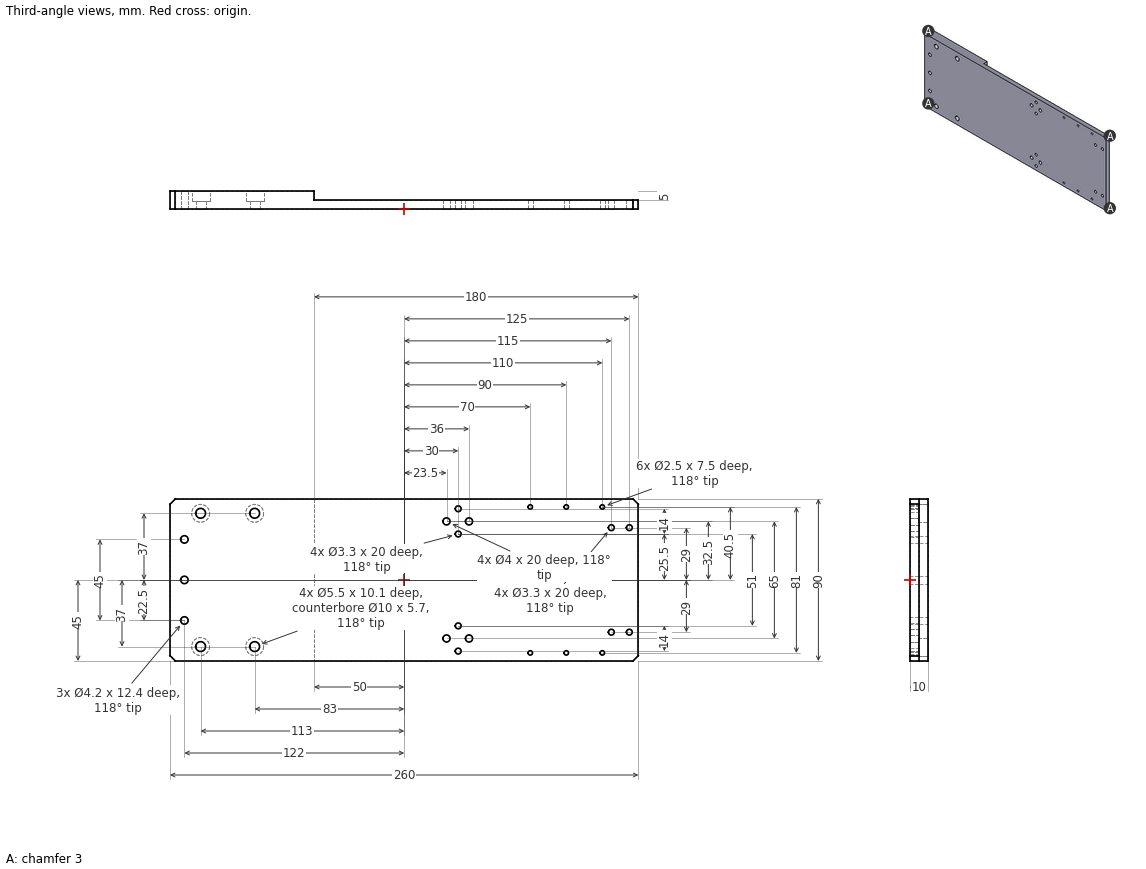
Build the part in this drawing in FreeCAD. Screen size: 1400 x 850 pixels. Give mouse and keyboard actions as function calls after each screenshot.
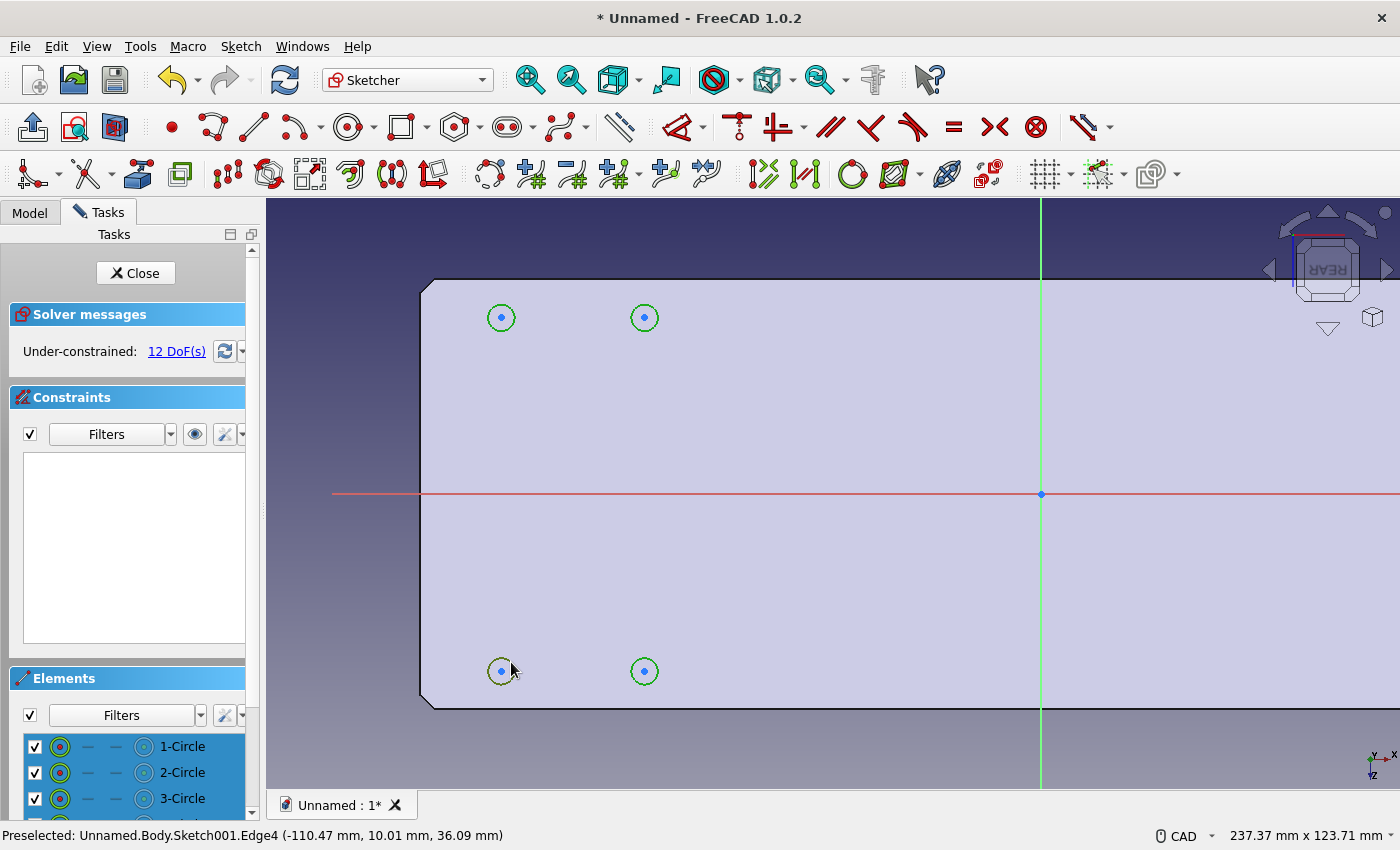
click(954, 128)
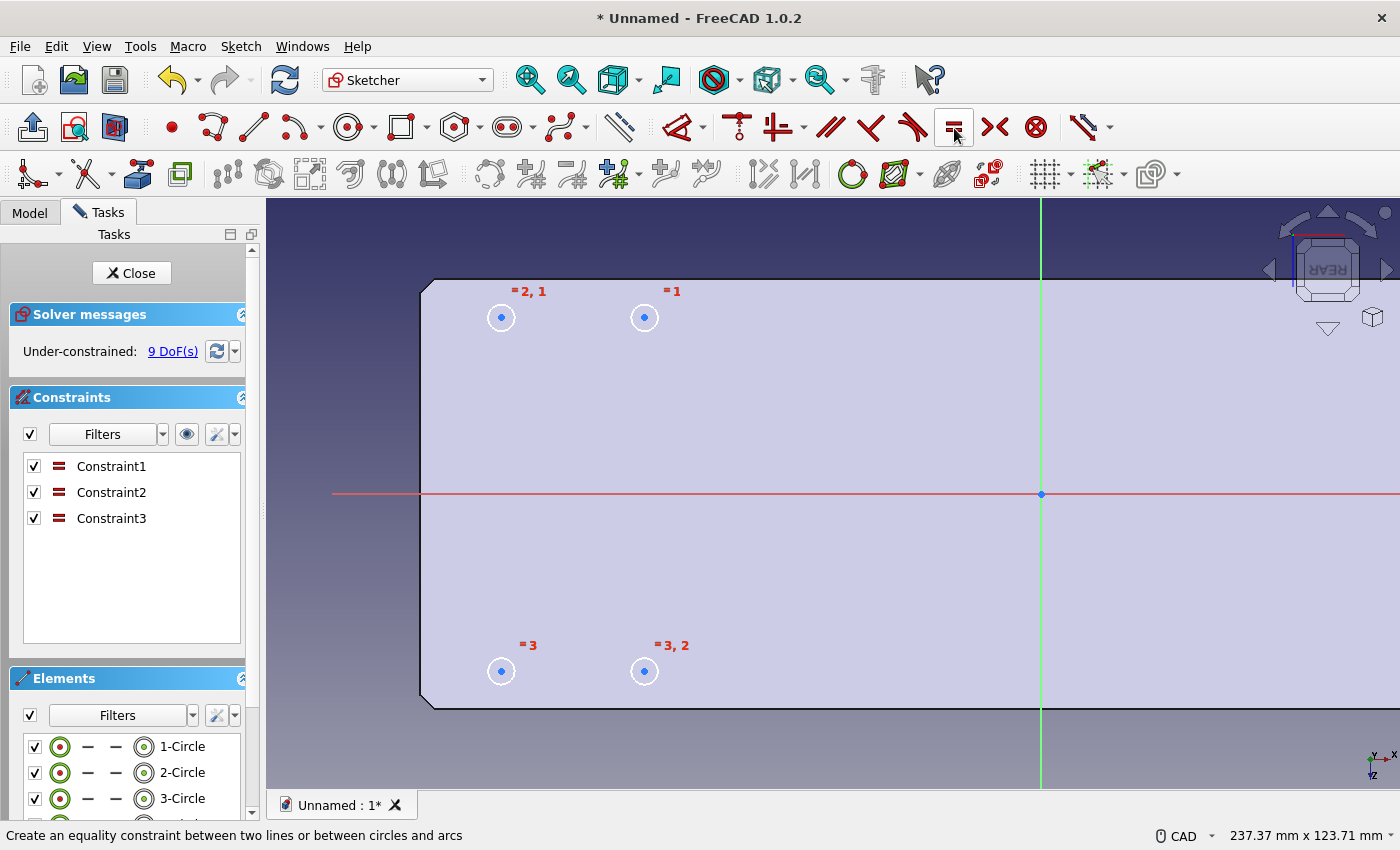
click(645, 318)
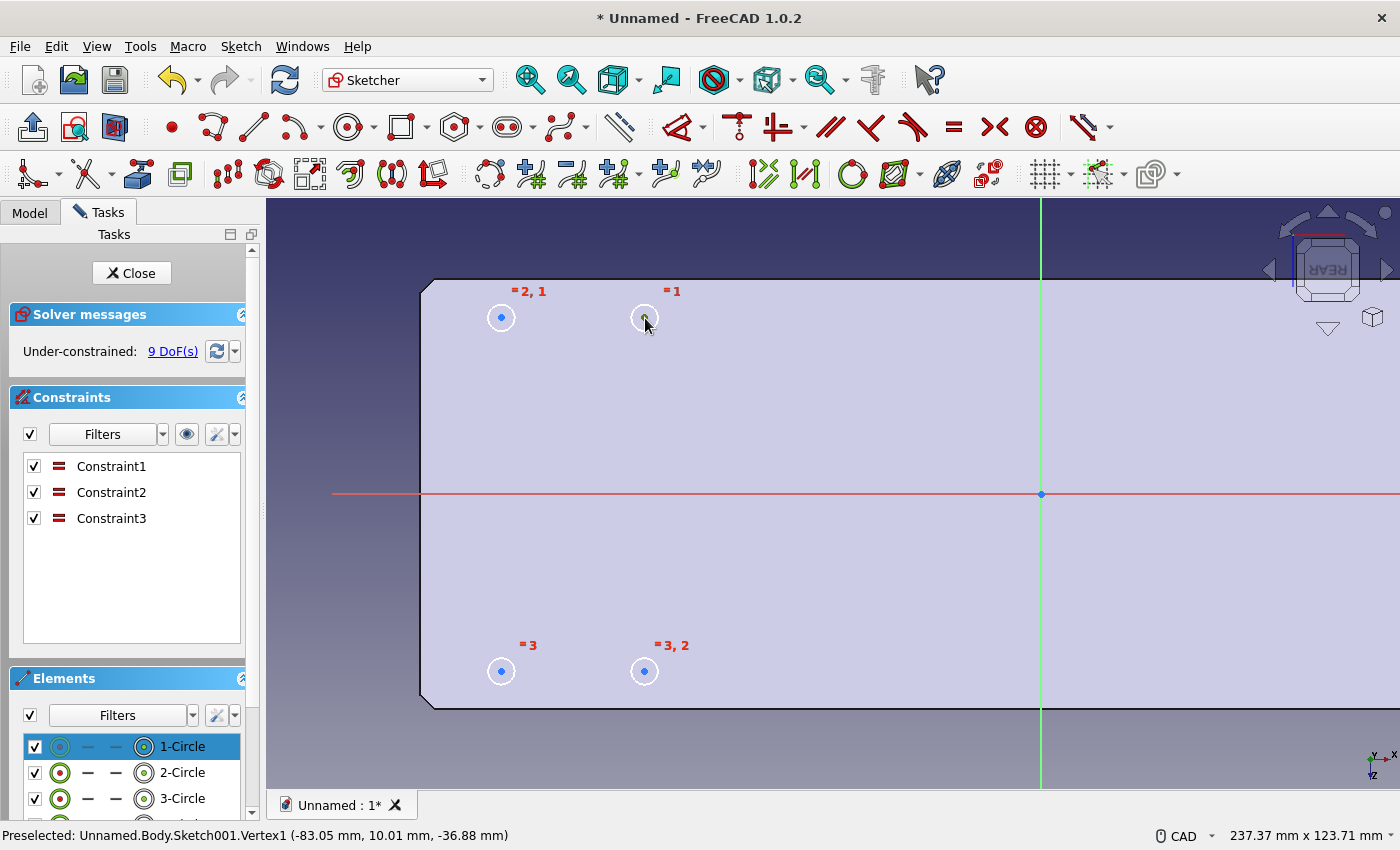
click(501, 318)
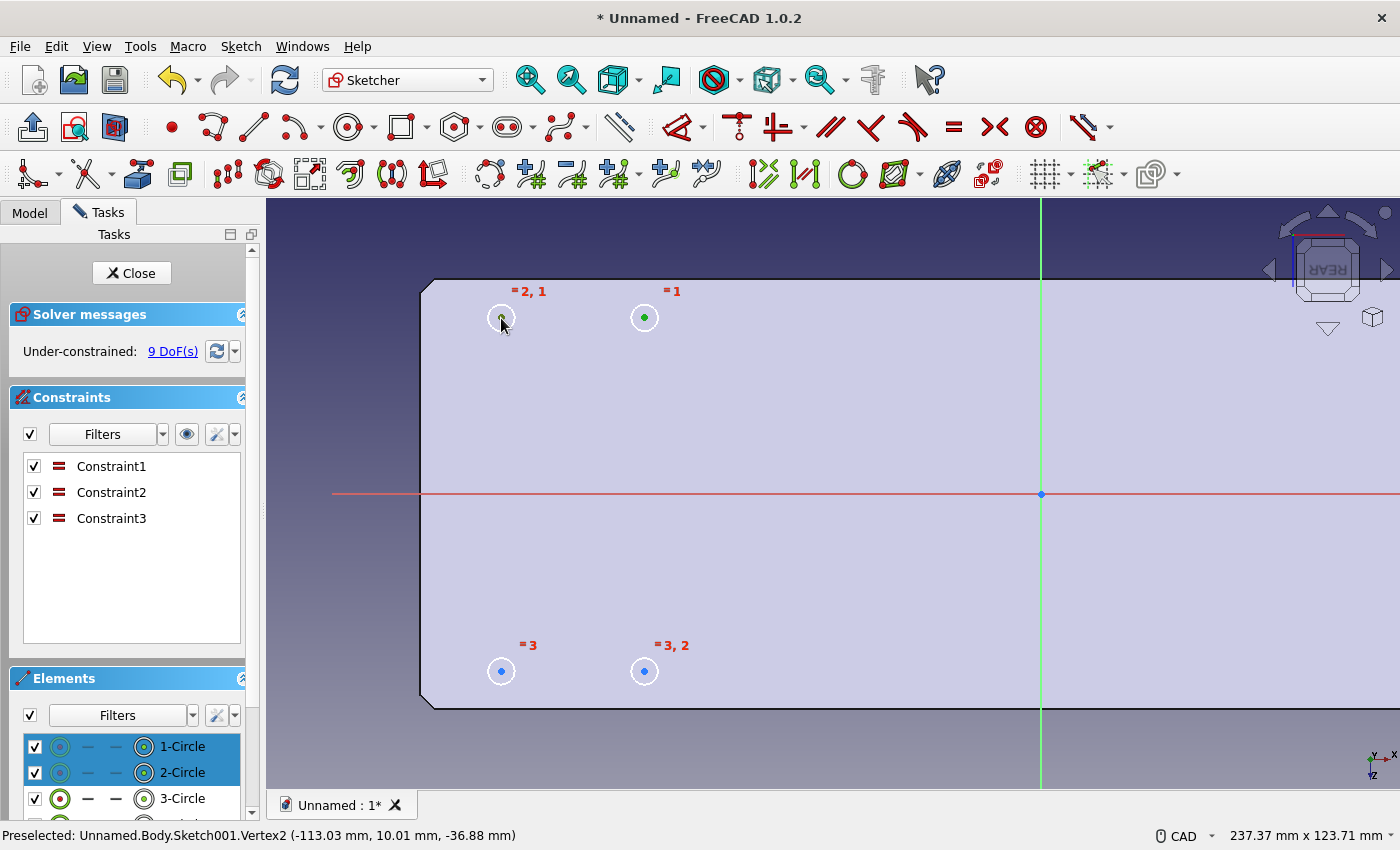
click(804, 128)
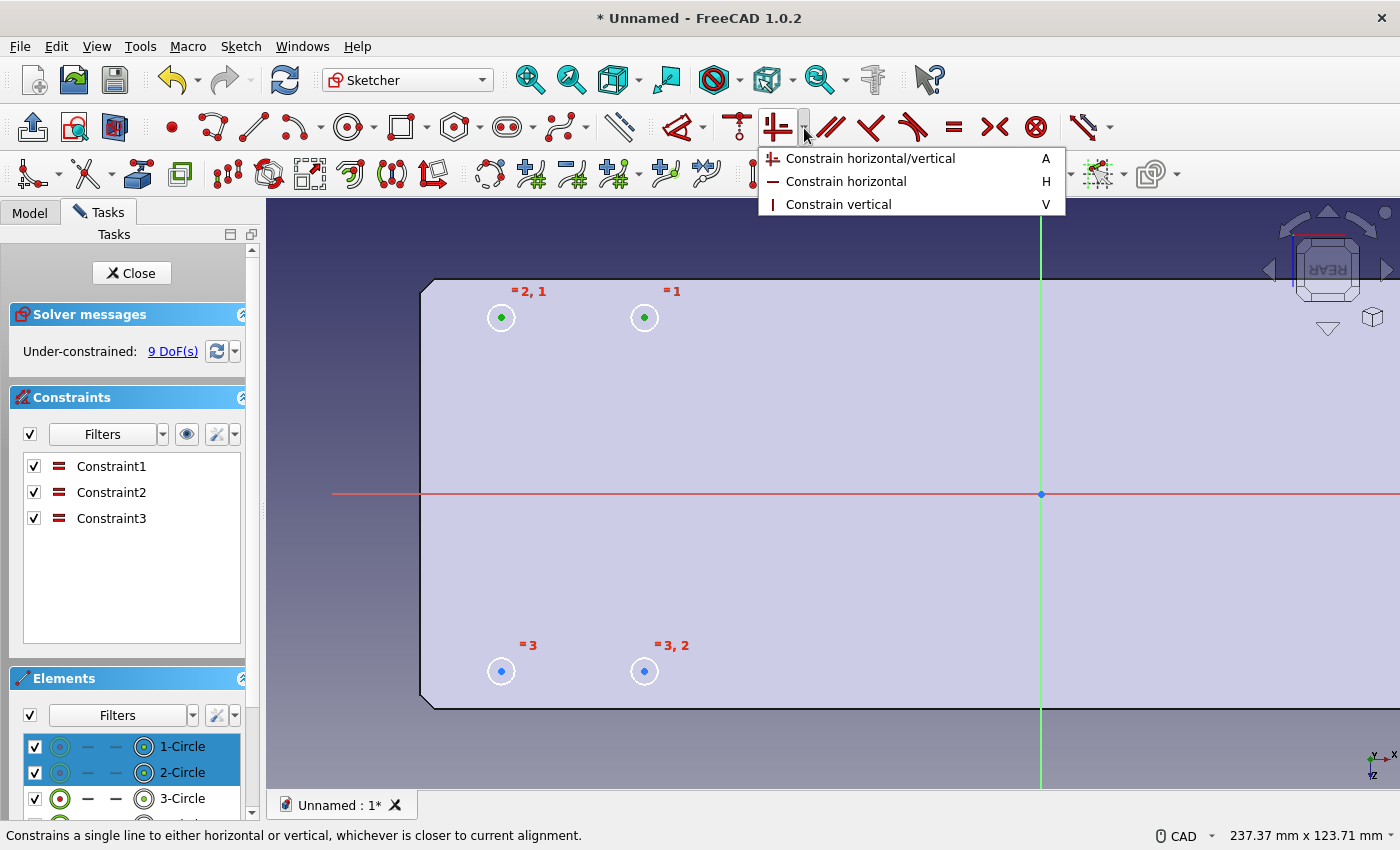
click(912, 182)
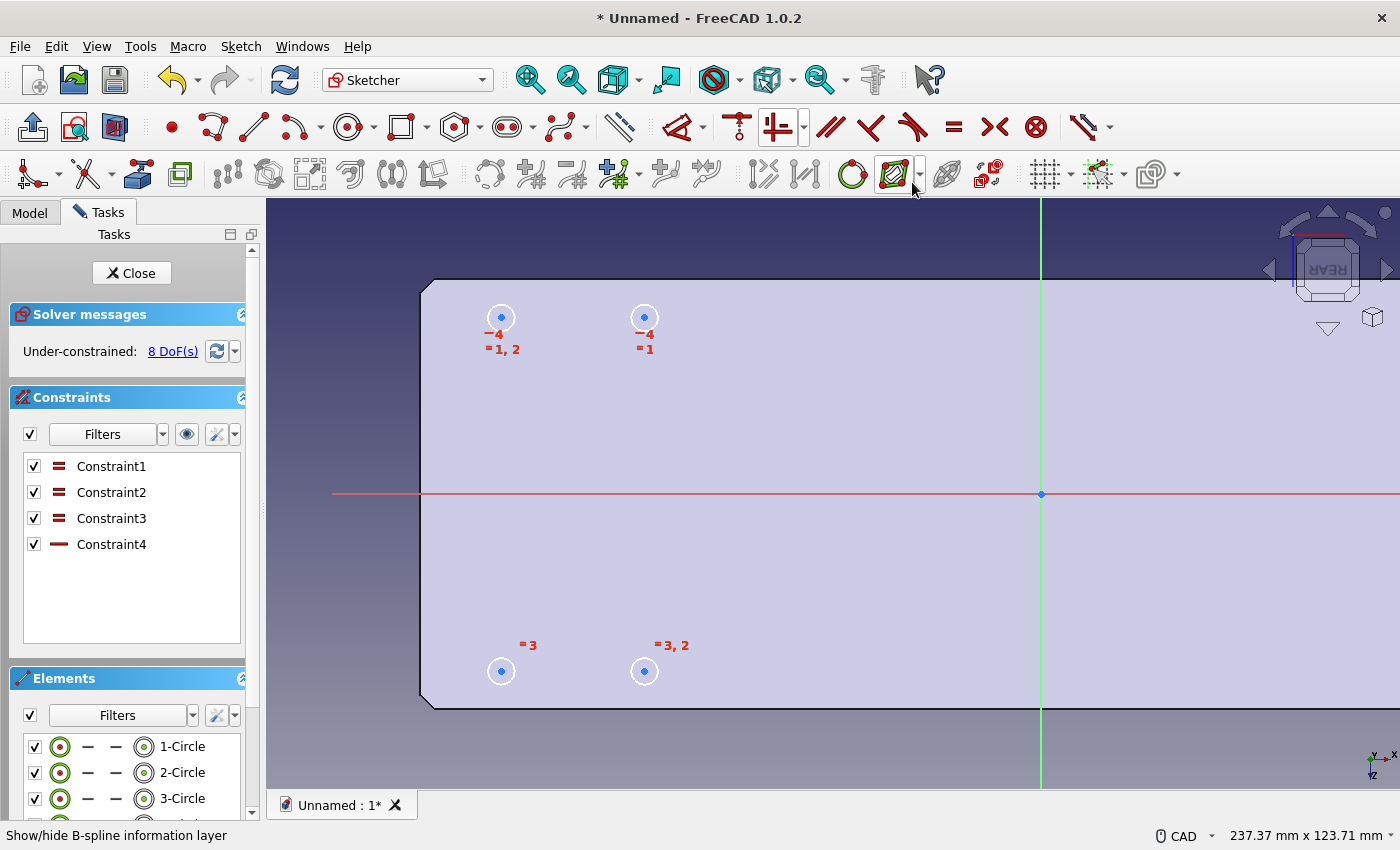
click(645, 318)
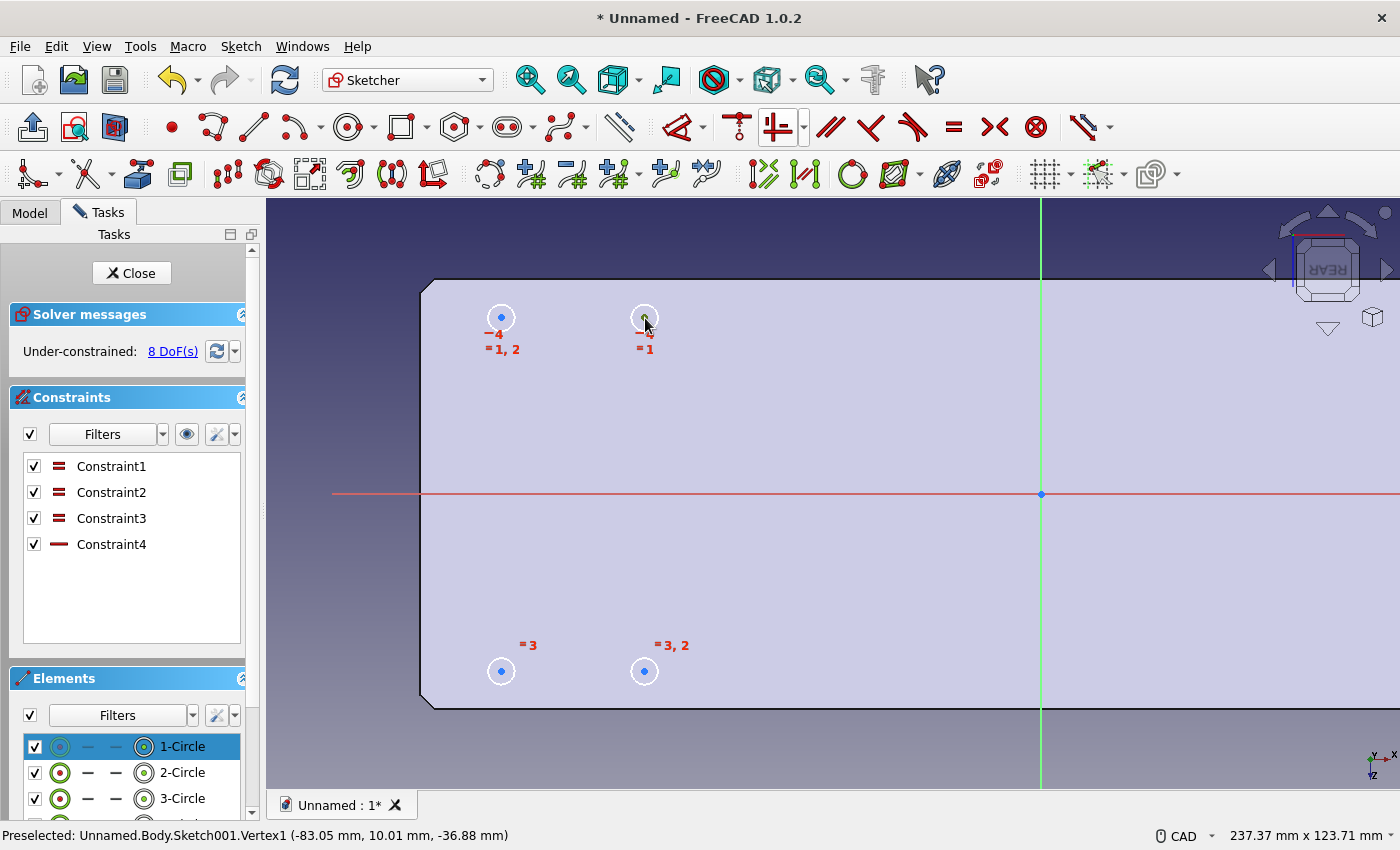
click(645, 671)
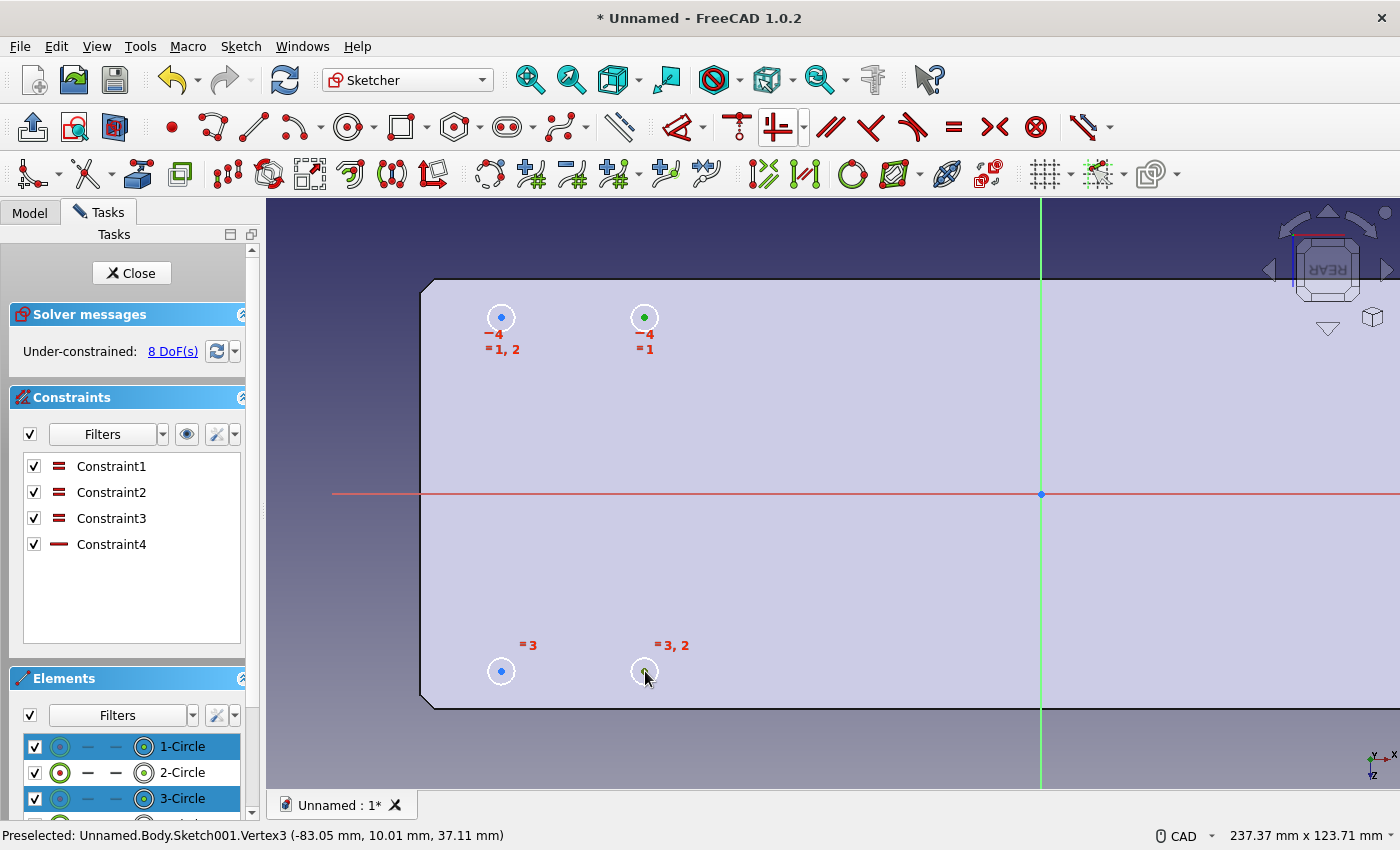
click(804, 128)